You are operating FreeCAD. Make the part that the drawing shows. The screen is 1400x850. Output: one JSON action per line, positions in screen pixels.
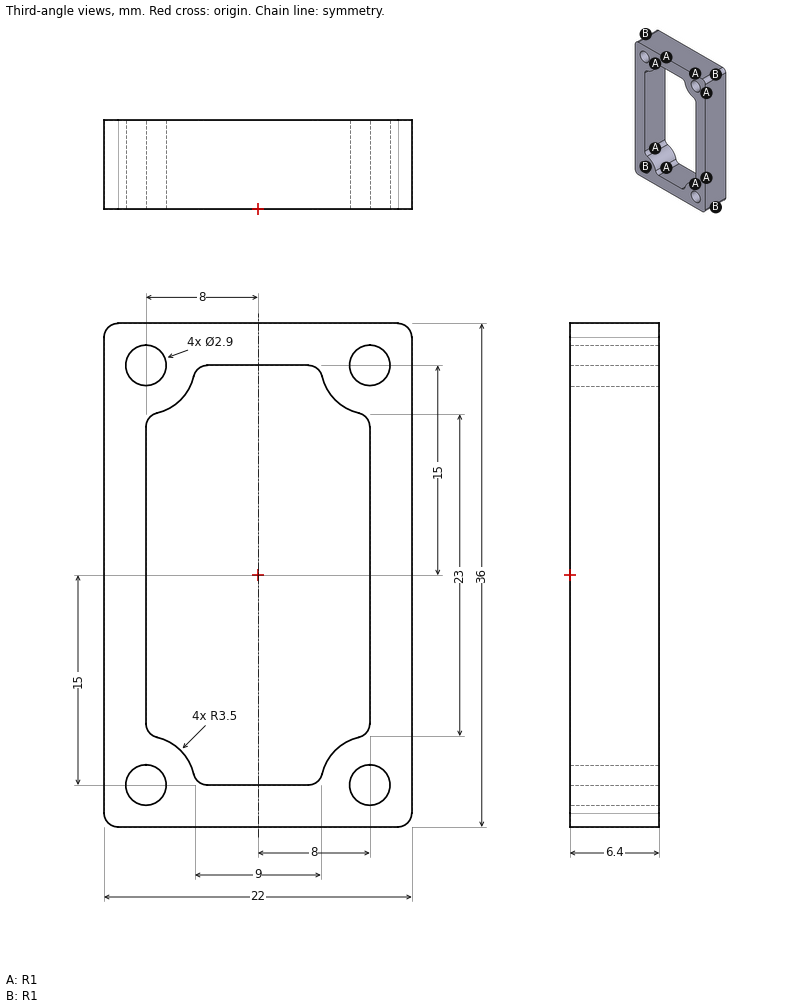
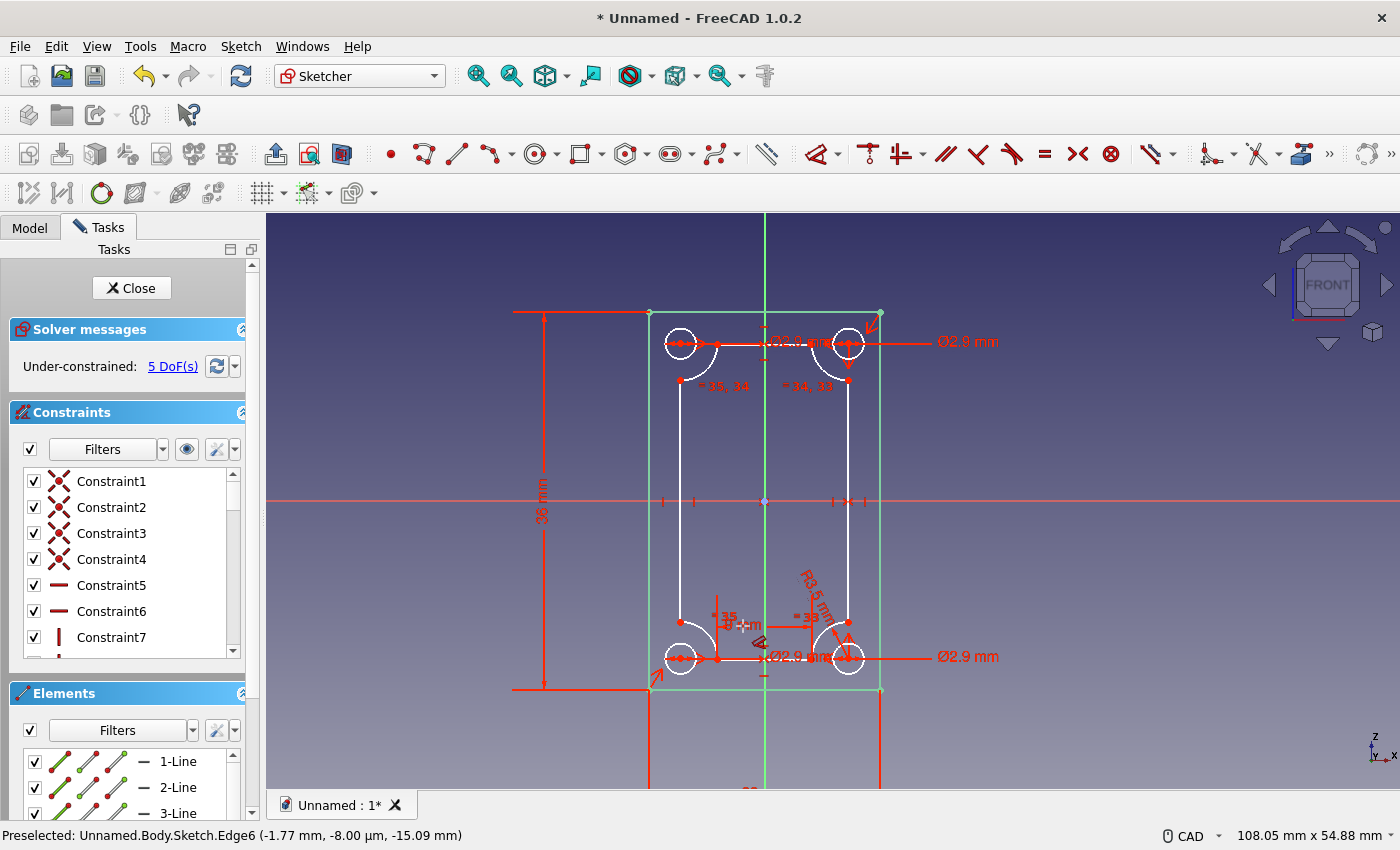
{"action": "left_click", "coordinate": [848, 550]}
{"action": "left_click", "coordinate": [814, 446]}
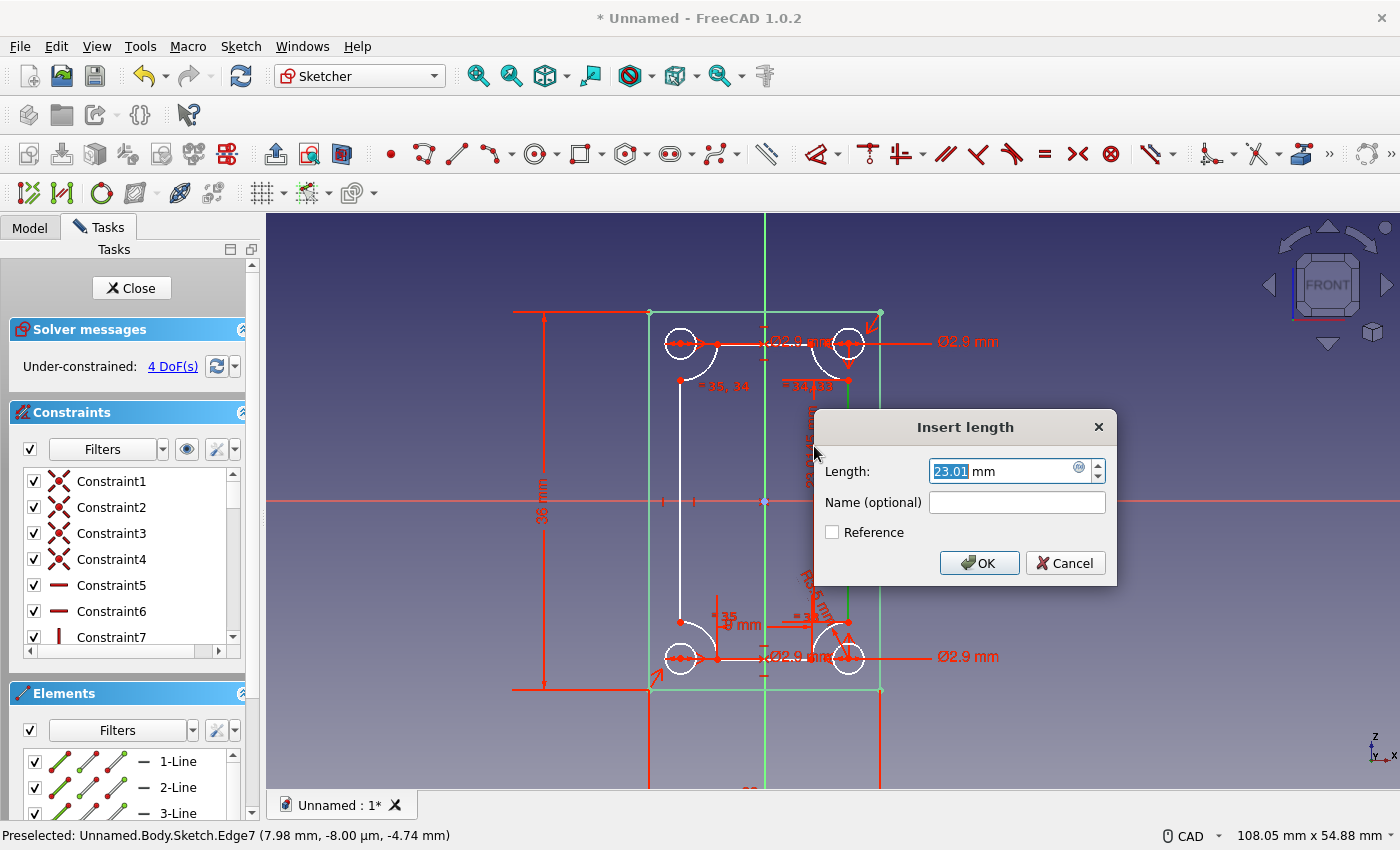
{"action": "type", "text": "23"}
{"action": "key", "text": "Return"}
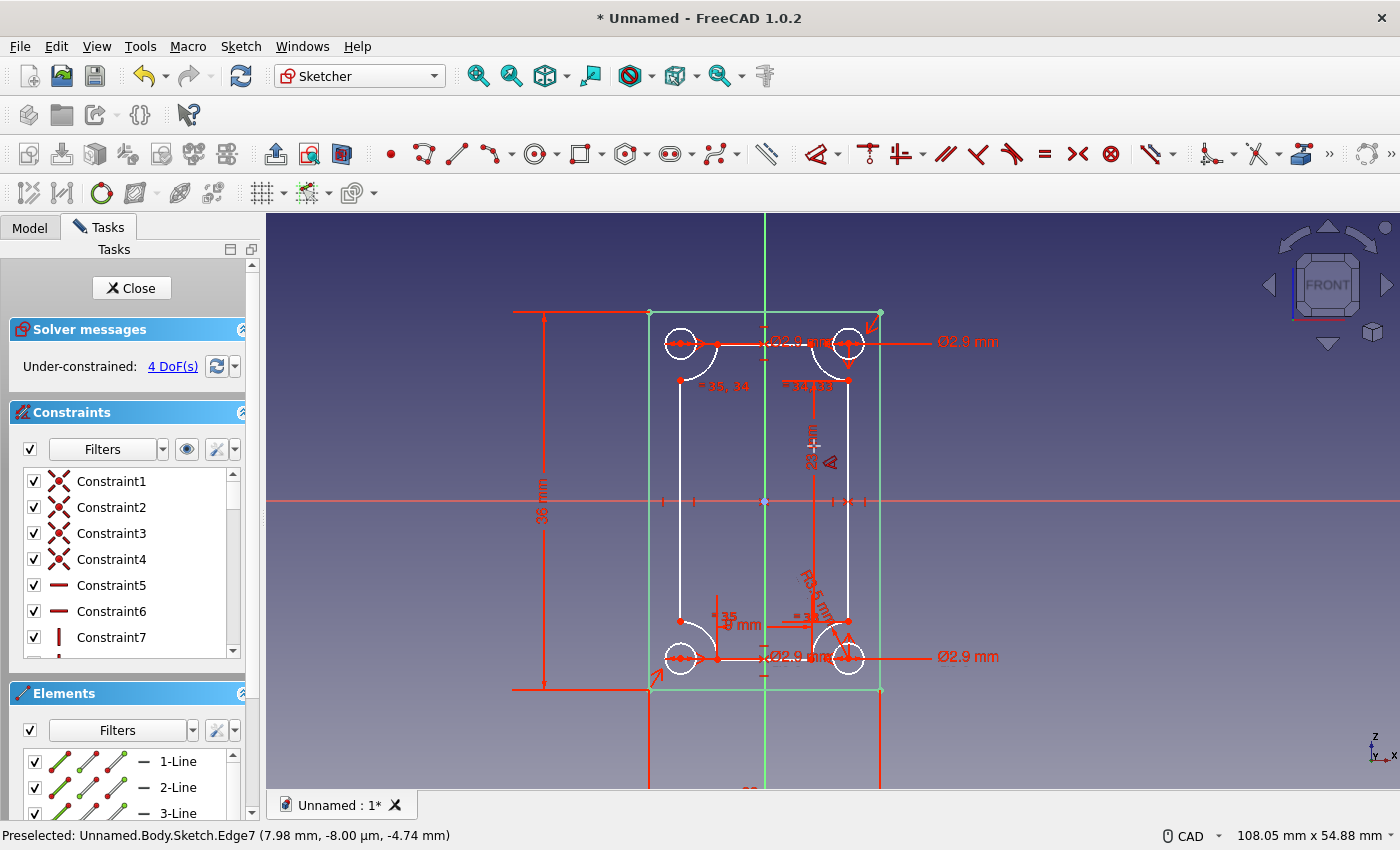
{"action": "left_click", "coordinate": [848, 622]}
{"action": "left_click", "coordinate": [806, 467]}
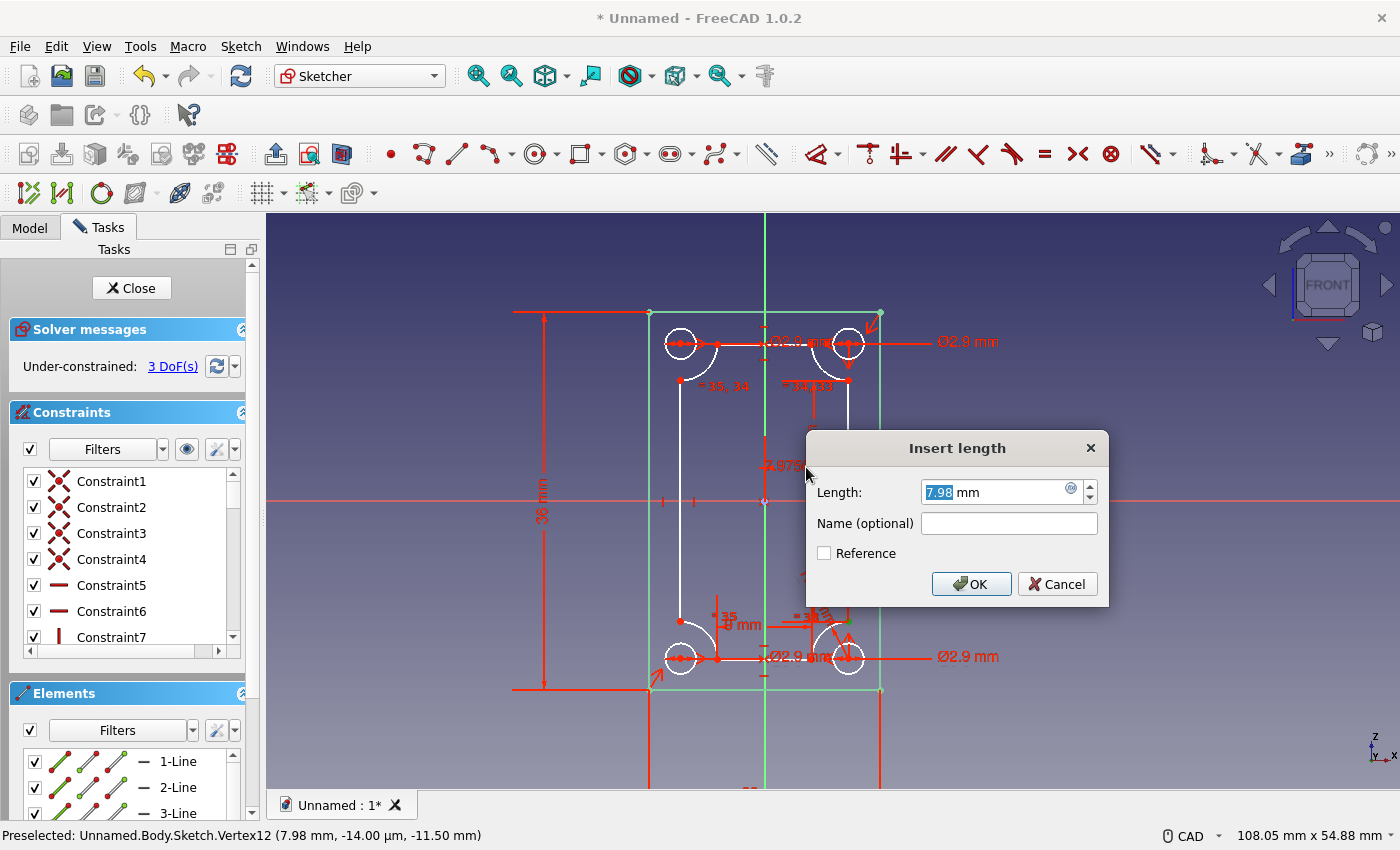
{"action": "type", "text": "8"}
{"action": "key", "text": "Return"}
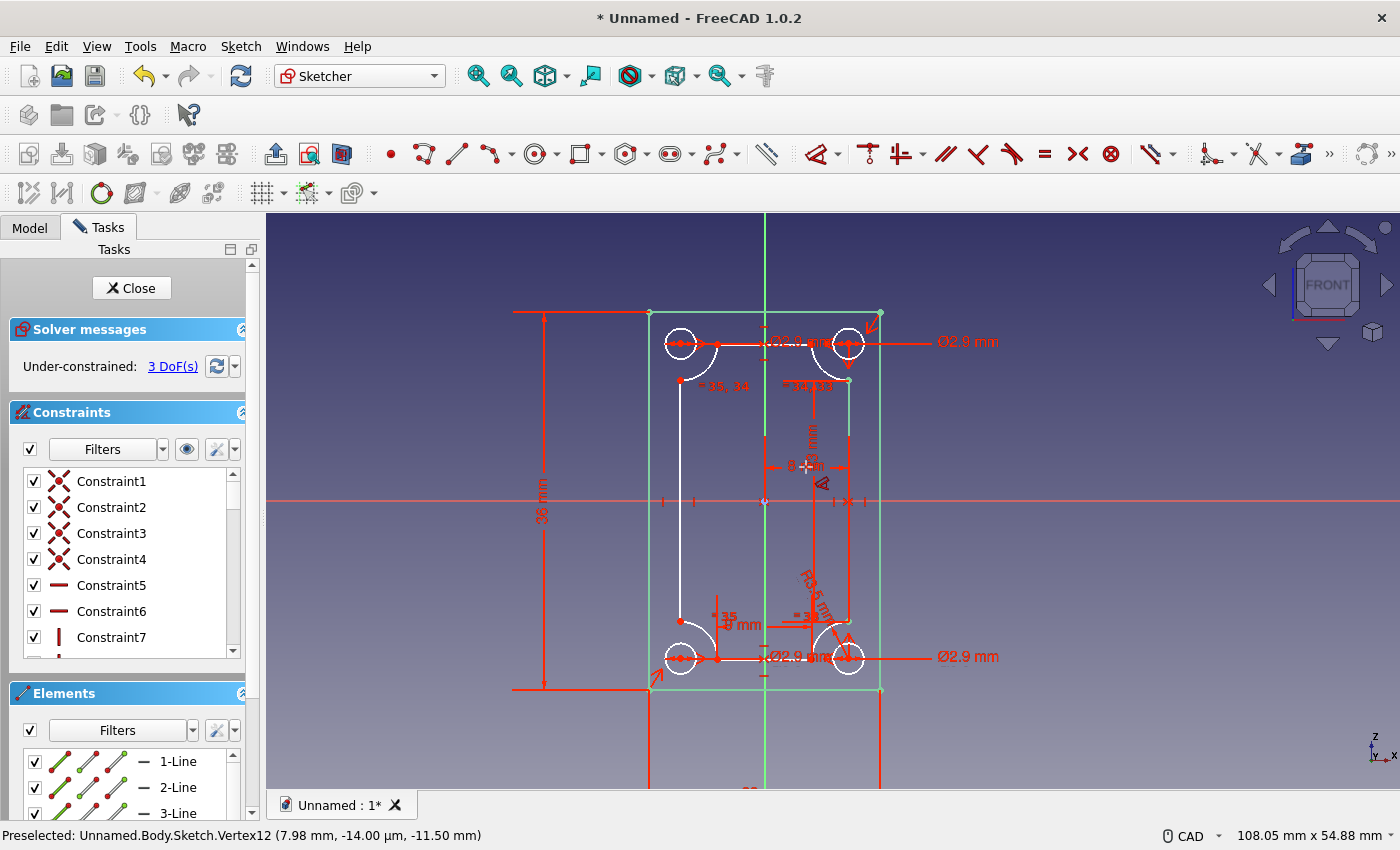
{"action": "left_click", "coordinate": [680, 381]}
{"action": "left_click", "coordinate": [722, 535]}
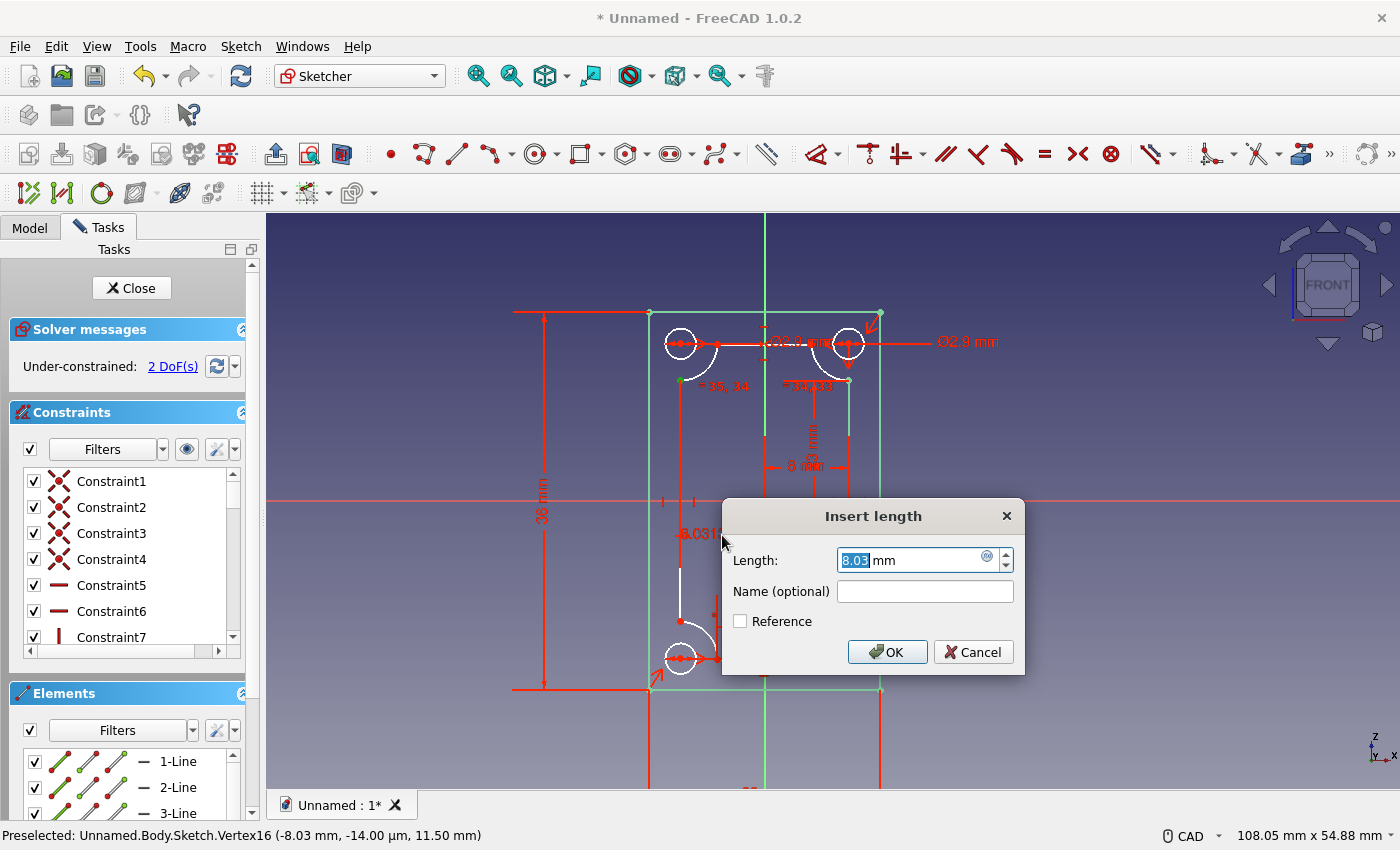
{"action": "type", "text": "8"}
{"action": "key", "text": "Return"}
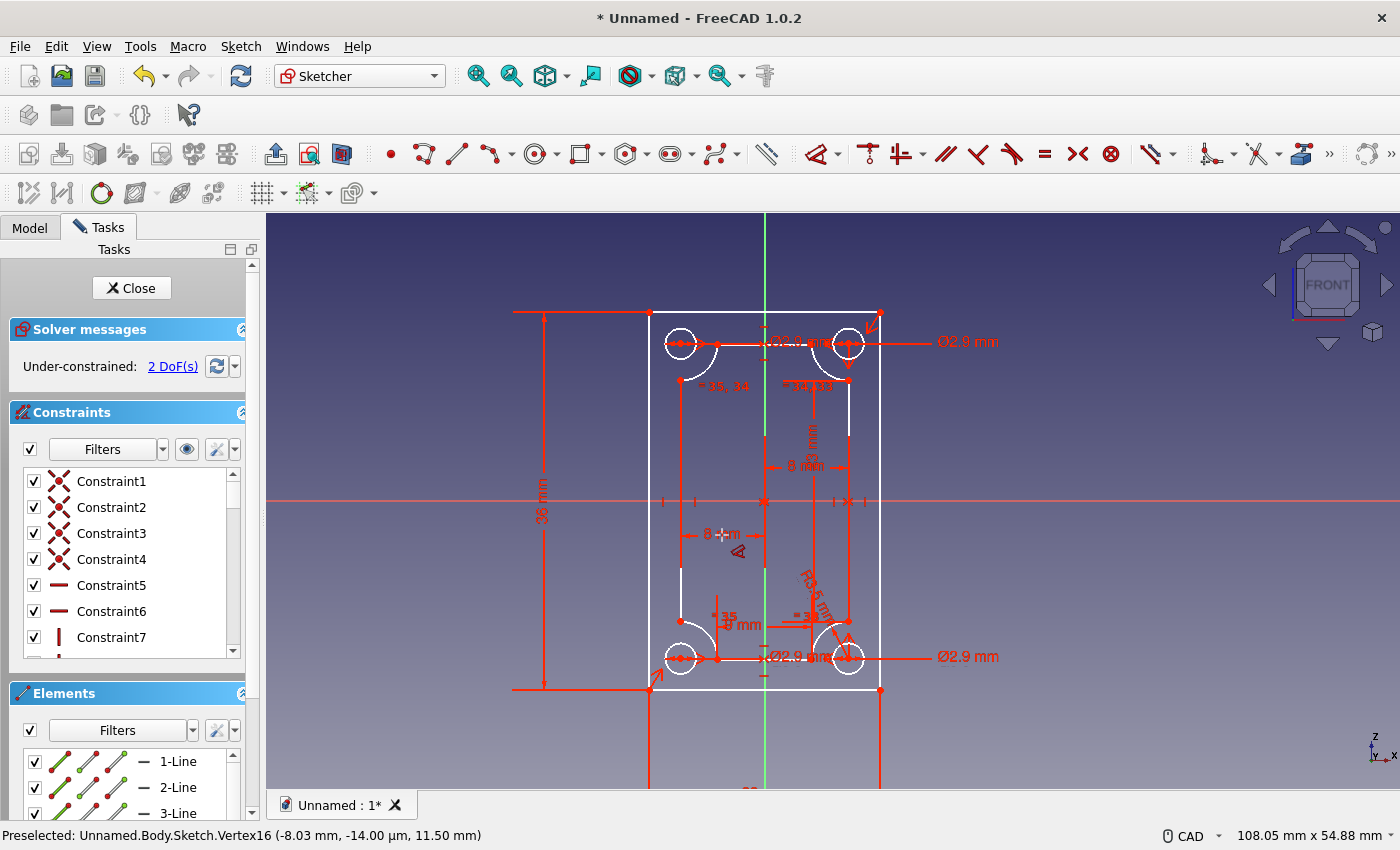
{"action": "left_click", "coordinate": [717, 660]}
{"action": "left_click", "coordinate": [799, 544]}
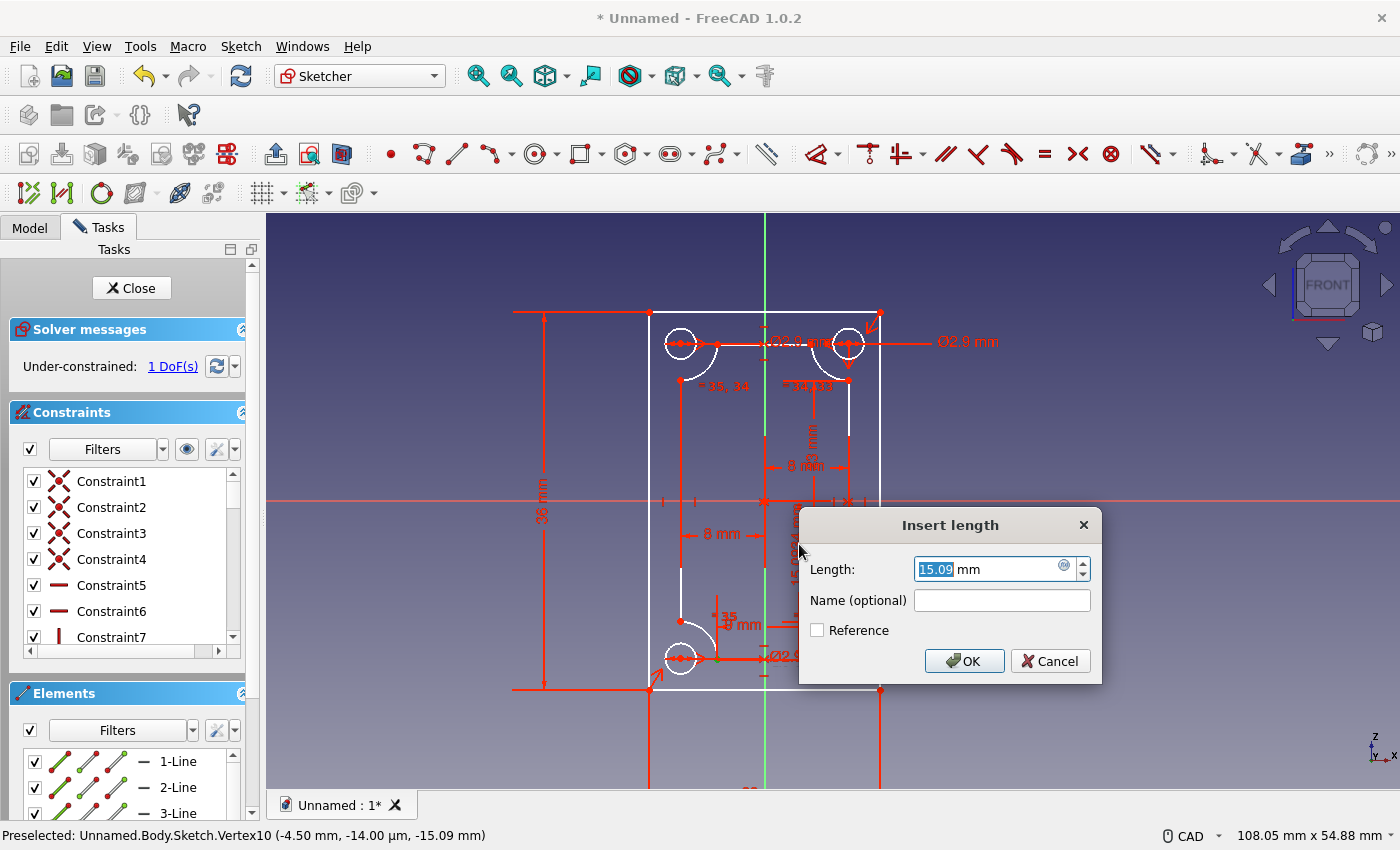
{"action": "type", "text": "15"}
{"action": "key", "text": "Return"}